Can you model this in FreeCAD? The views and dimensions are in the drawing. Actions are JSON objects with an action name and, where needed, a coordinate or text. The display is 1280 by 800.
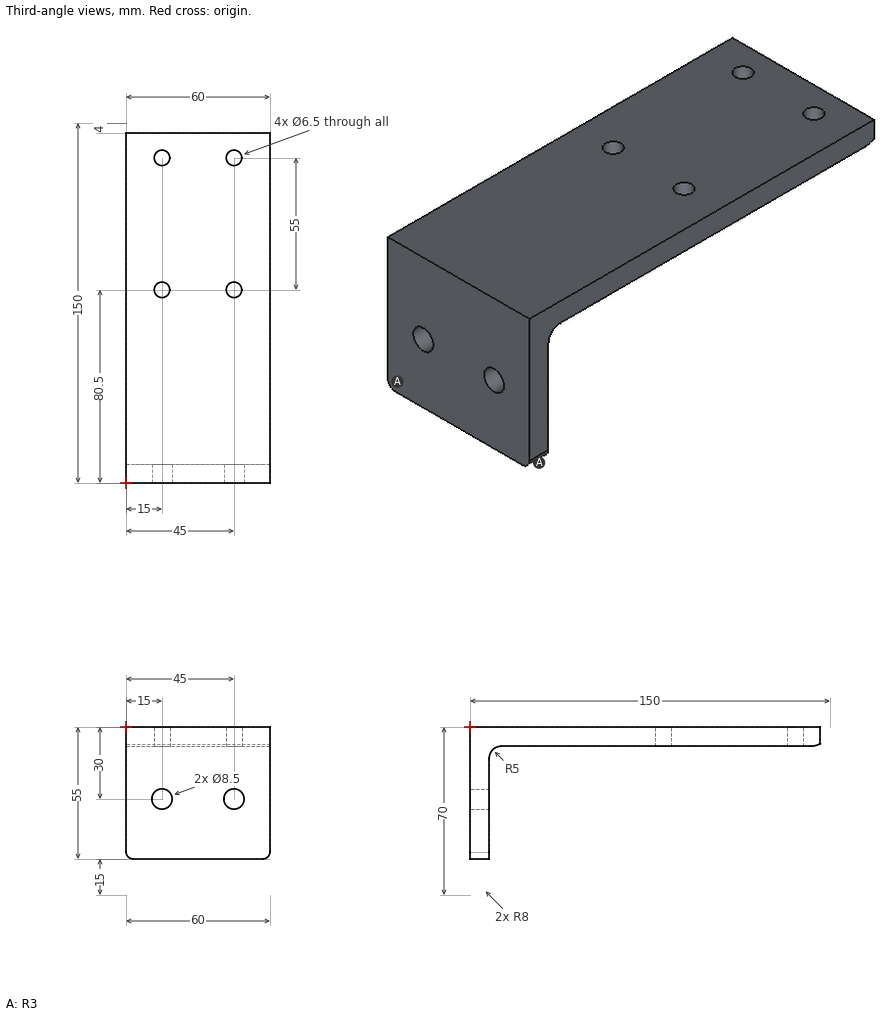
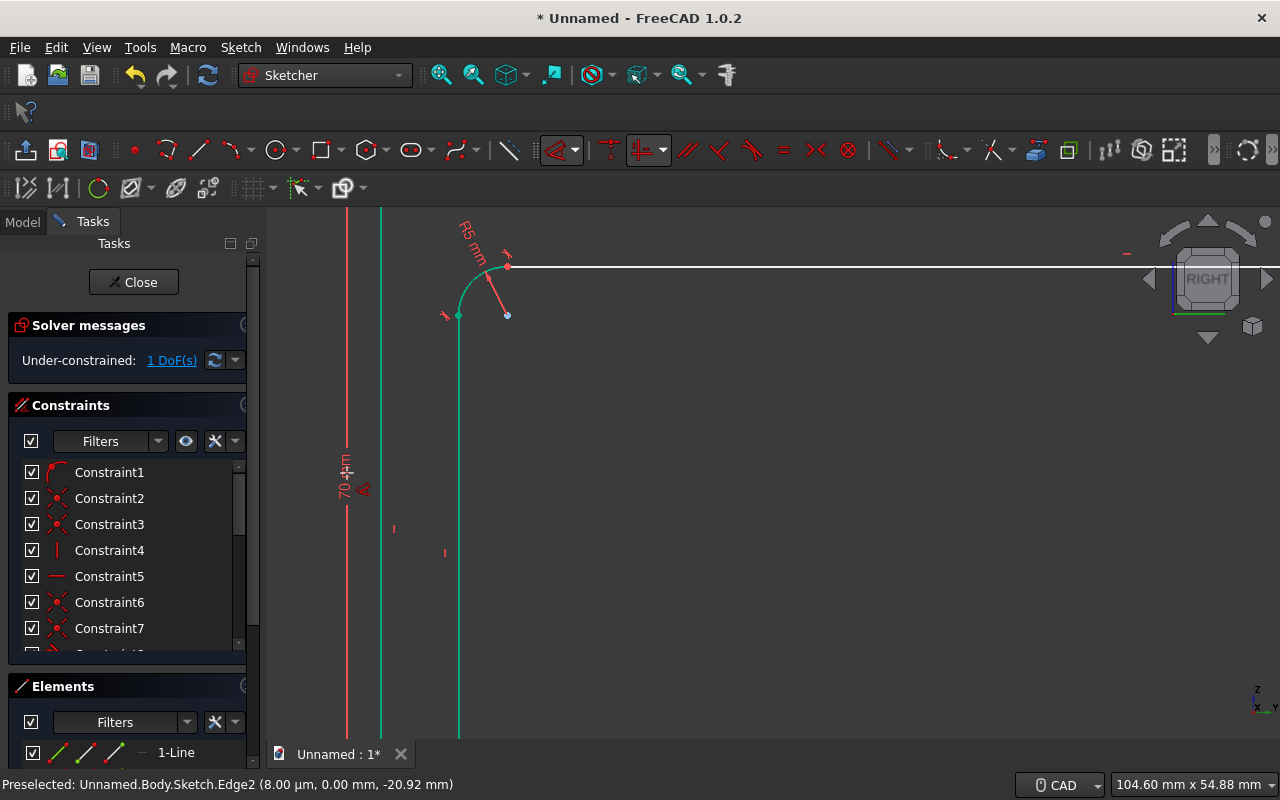
{"action": "scroll", "coordinate": [470, 441], "scroll_direction": "down", "scroll_amount": 5}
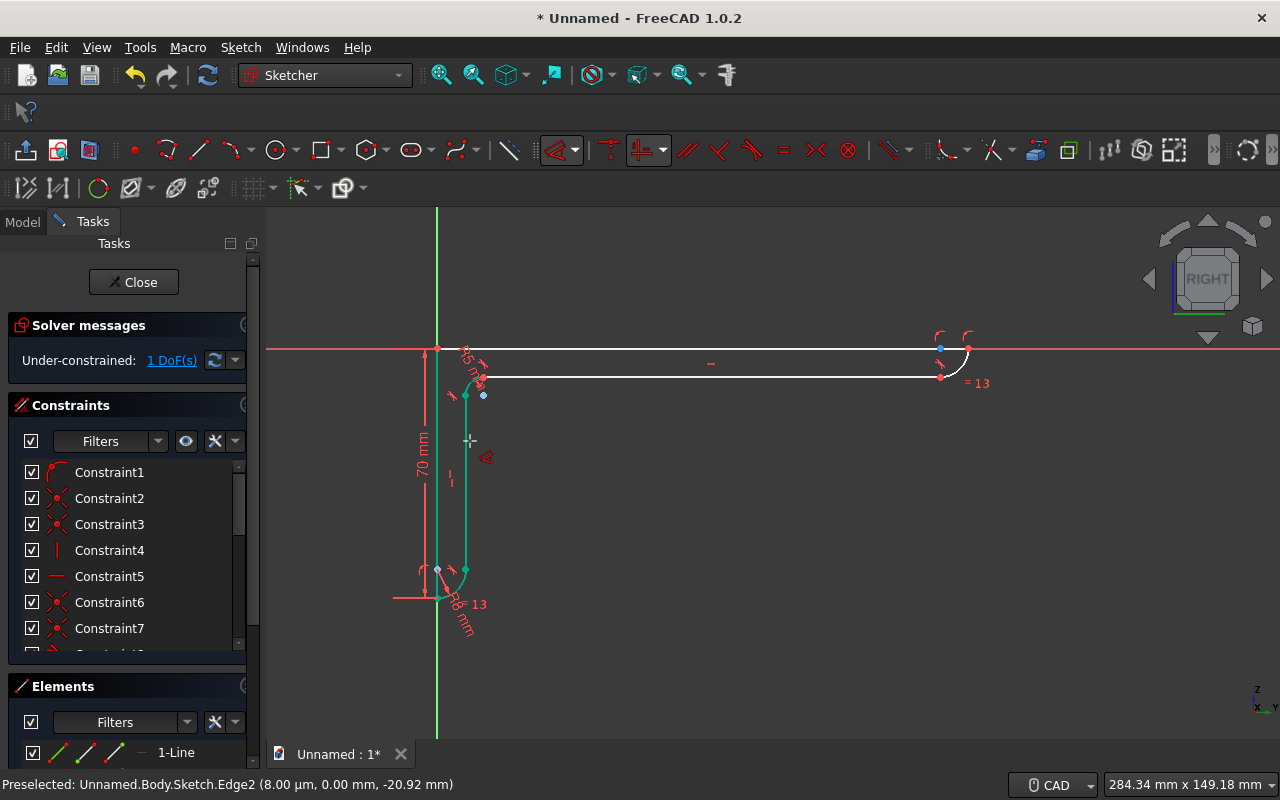
{"action": "left_click", "coordinate": [809, 349]}
{"action": "left_click", "coordinate": [703, 315]}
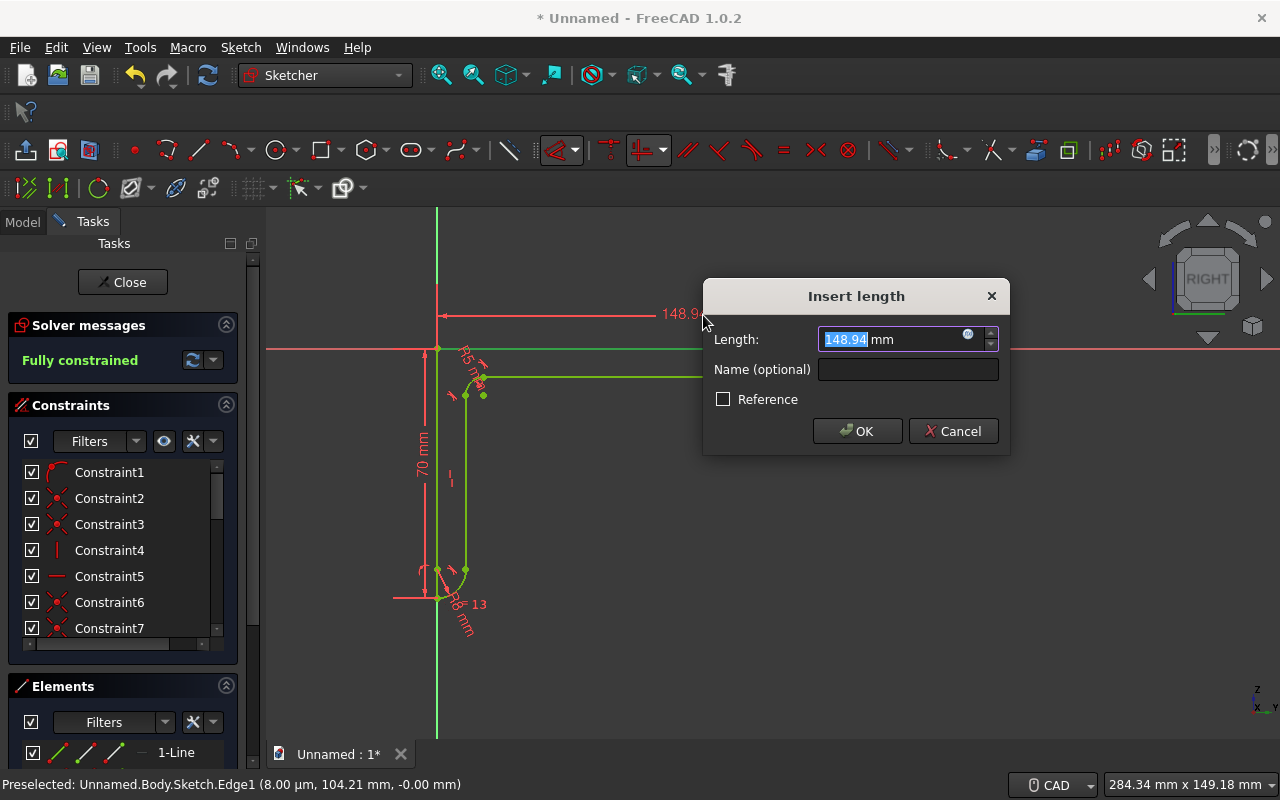
{"action": "type", "text": "150"}
{"action": "key", "text": "Return"}
{"action": "key", "text": "Escape"}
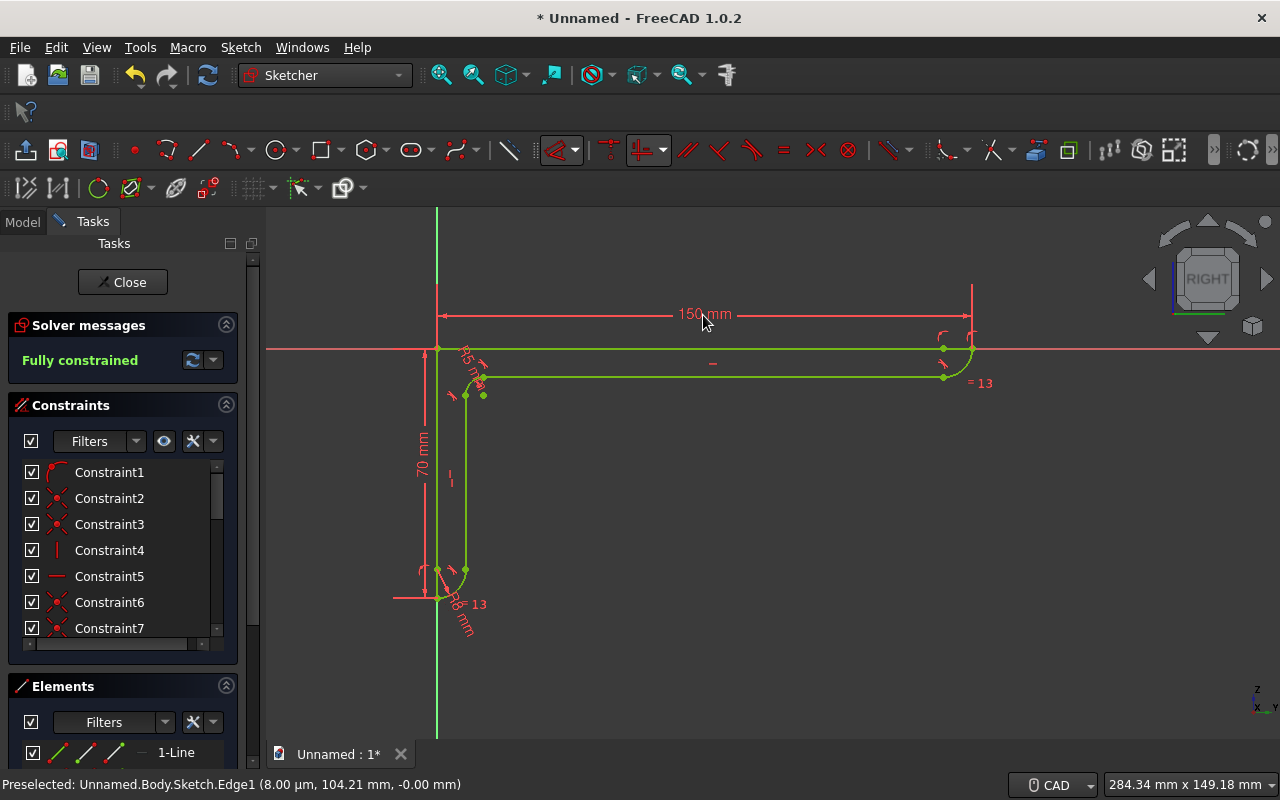
{"action": "left_click", "coordinate": [123, 282]}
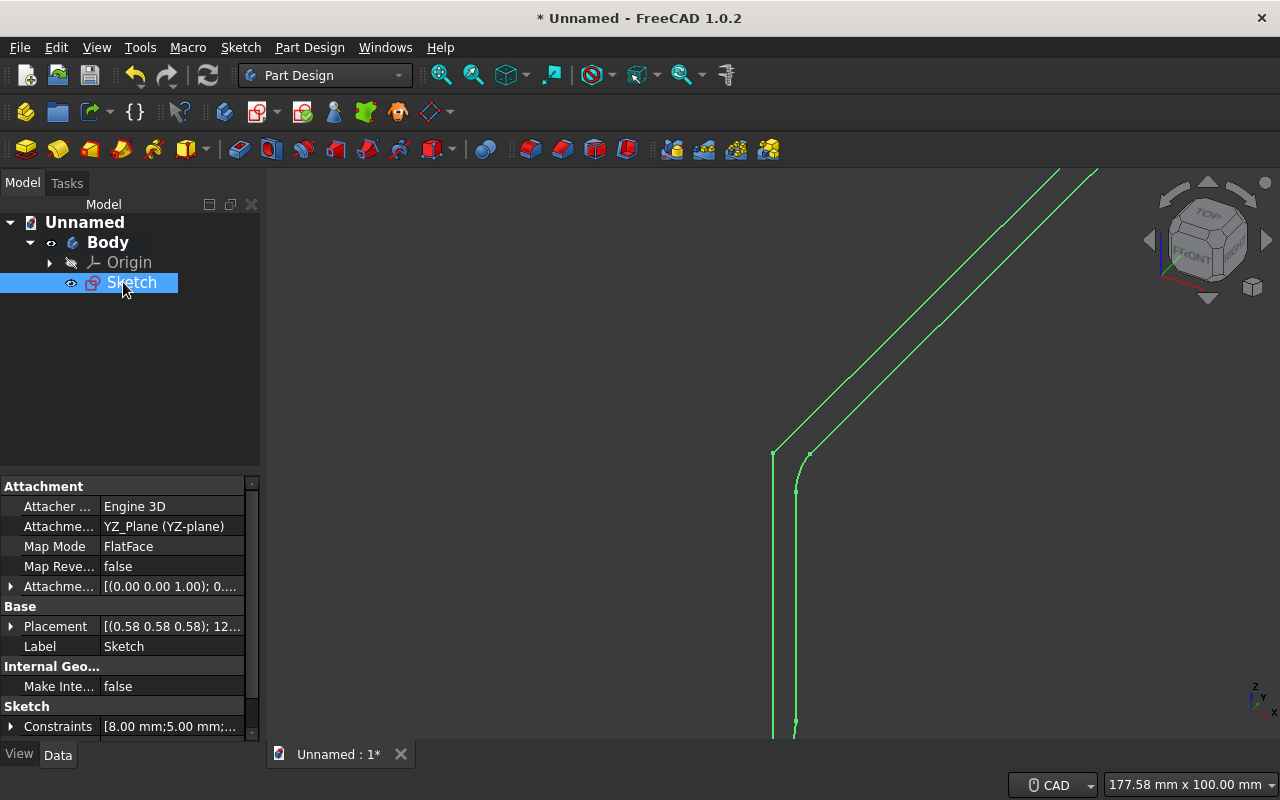
{"action": "left_click", "coordinate": [26, 150]}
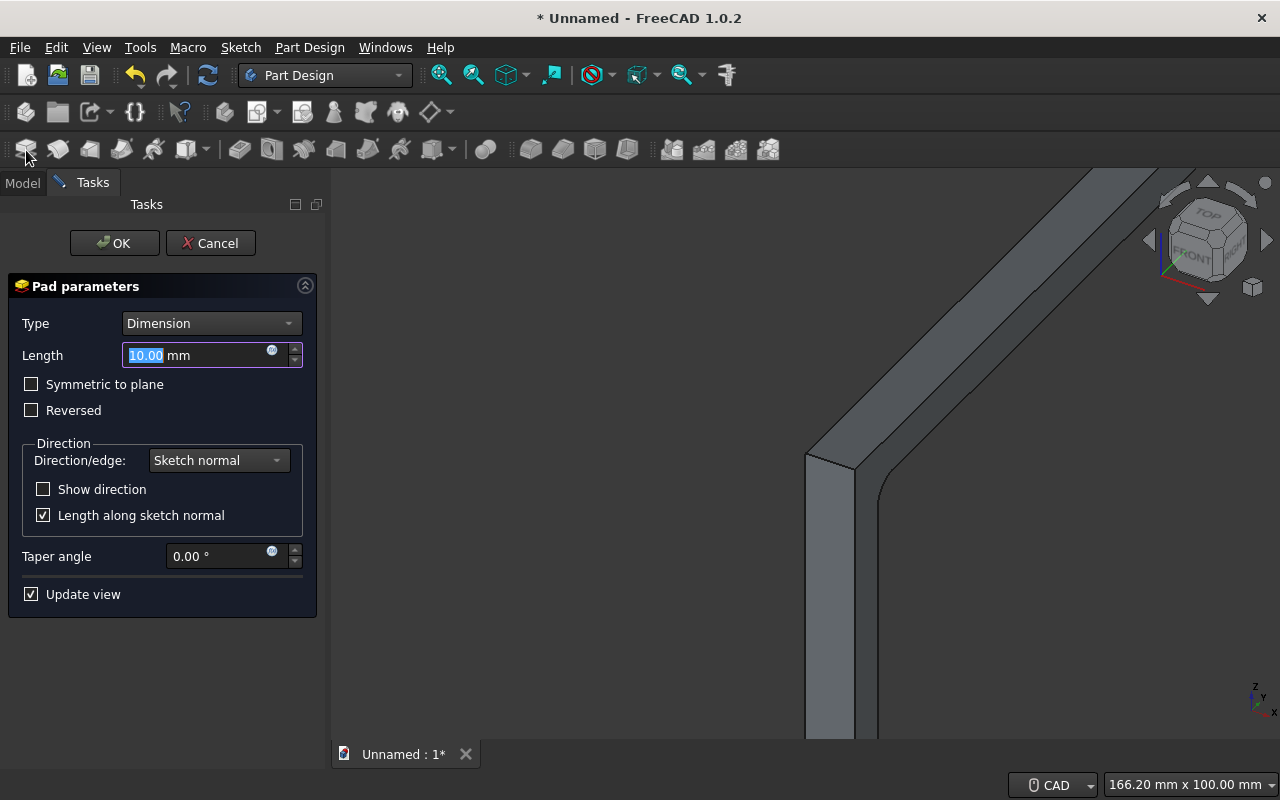
{"action": "type", "text": "60"}
{"action": "key", "text": "Tab"}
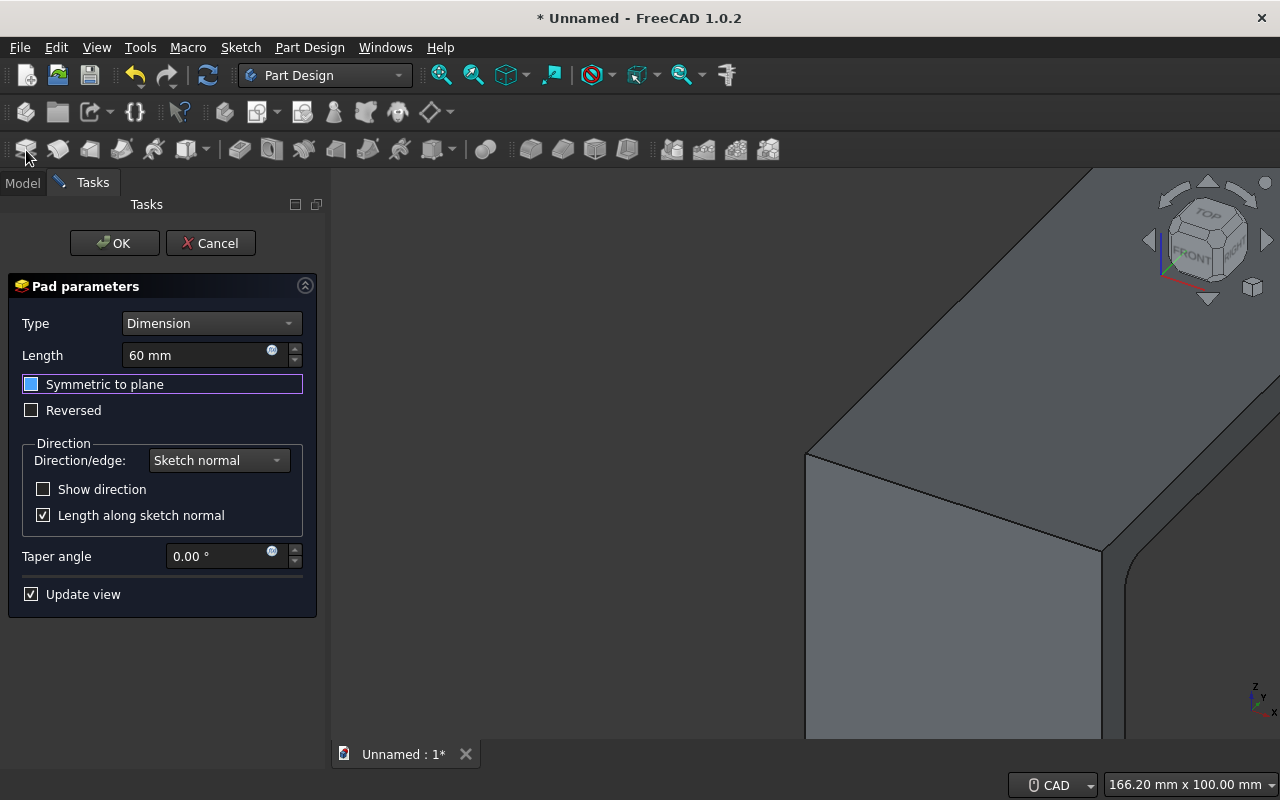
{"action": "left_click", "coordinate": [115, 243]}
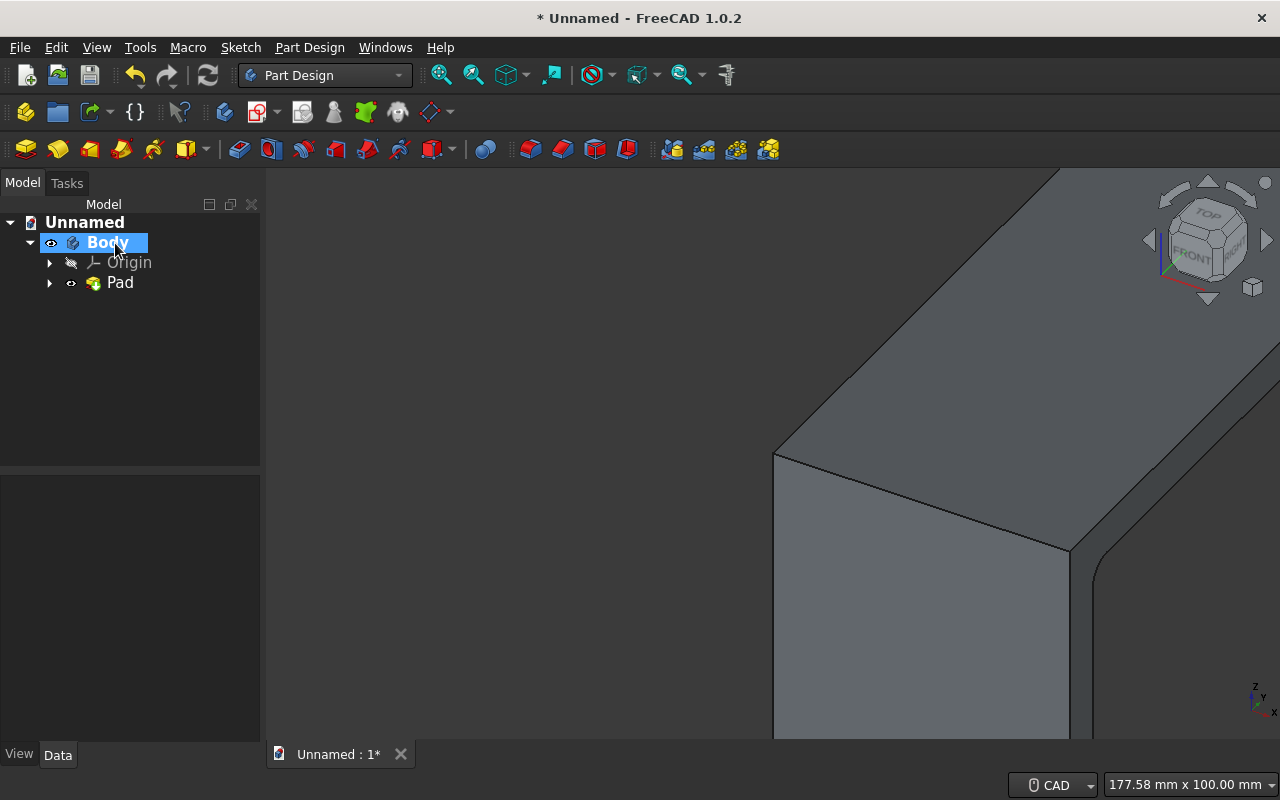
{"action": "key", "text": "v f"}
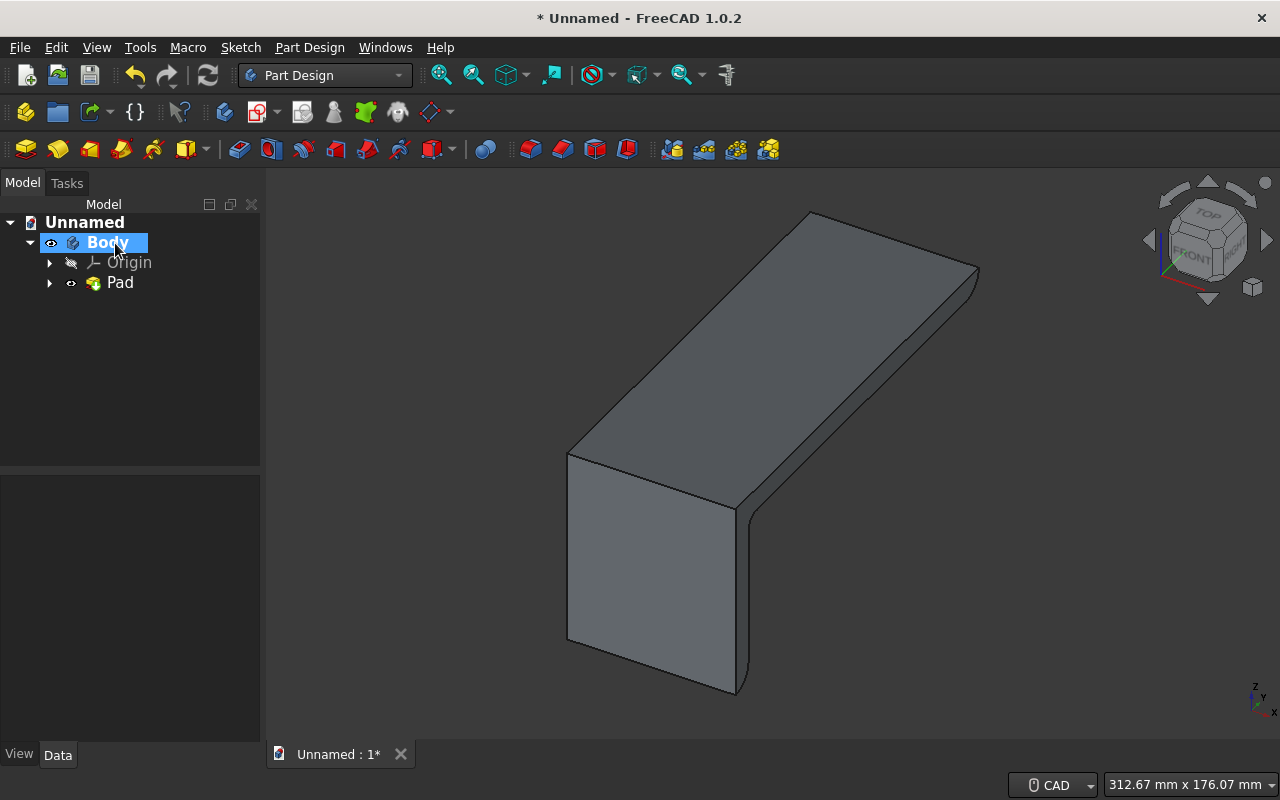
{"action": "left_click", "coordinate": [651, 573]}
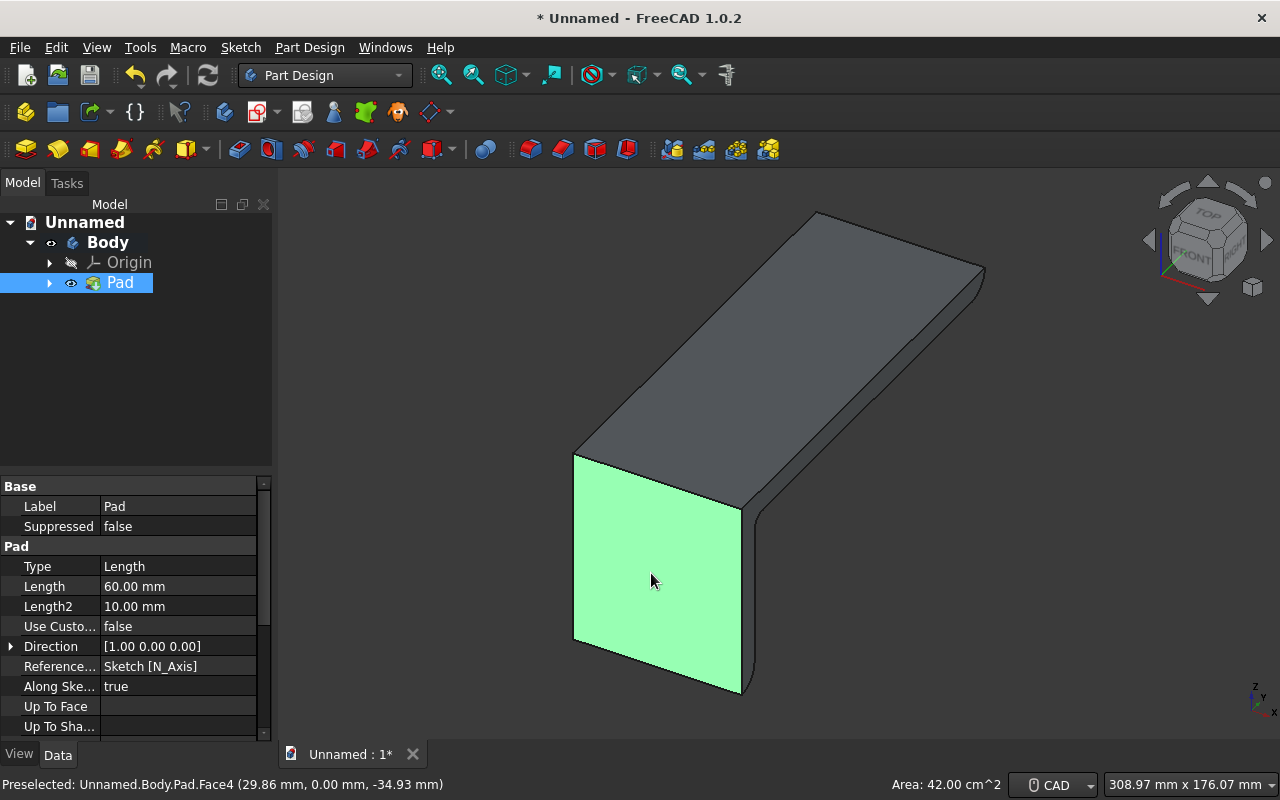
{"action": "left_click", "coordinate": [258, 112]}